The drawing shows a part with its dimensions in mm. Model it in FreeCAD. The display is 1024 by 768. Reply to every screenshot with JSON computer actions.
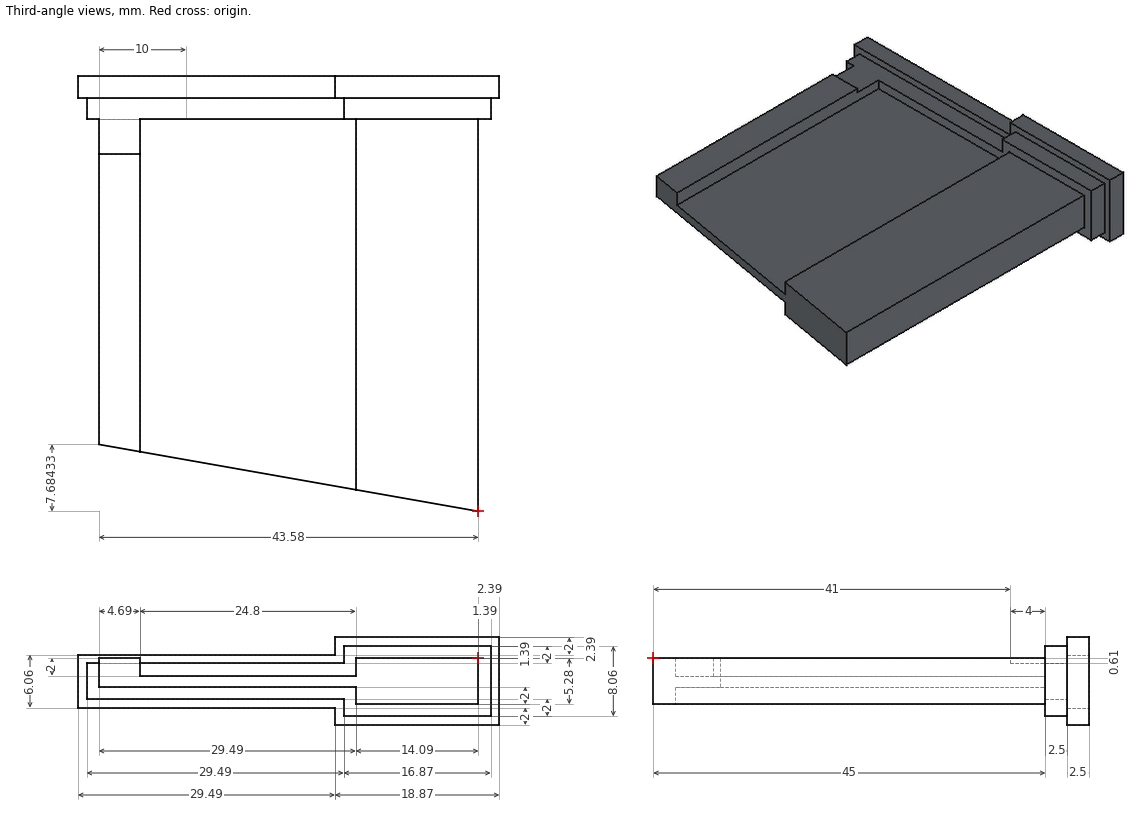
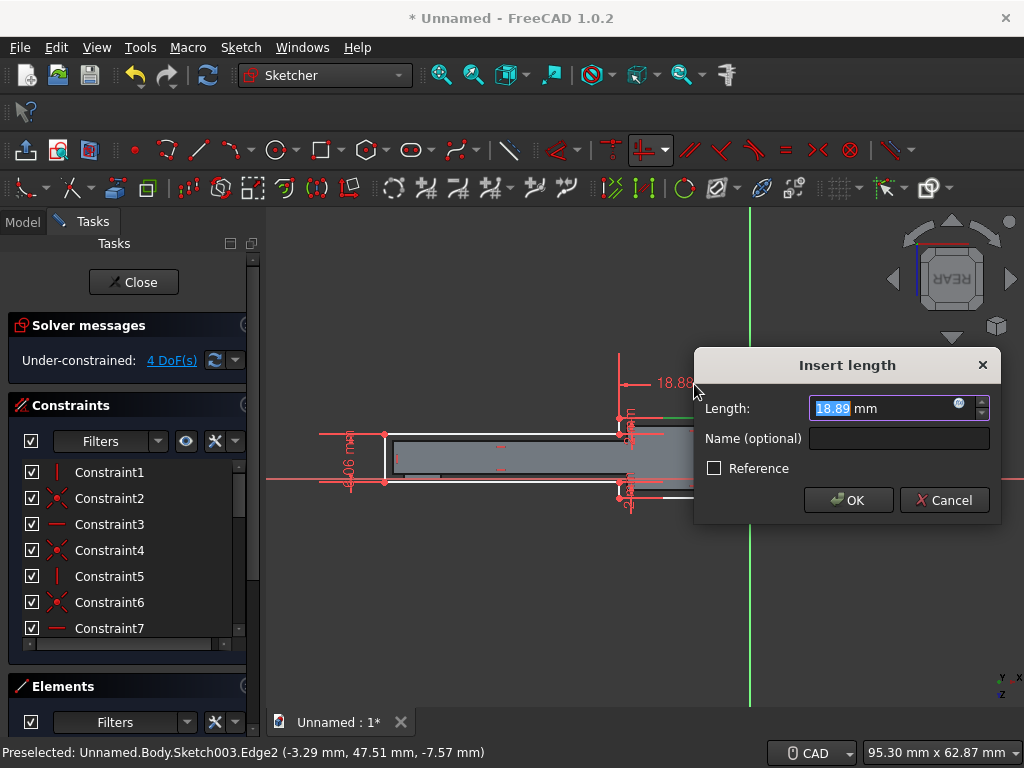
{"action": "type", "text": "18.87"}
{"action": "key", "text": "Return"}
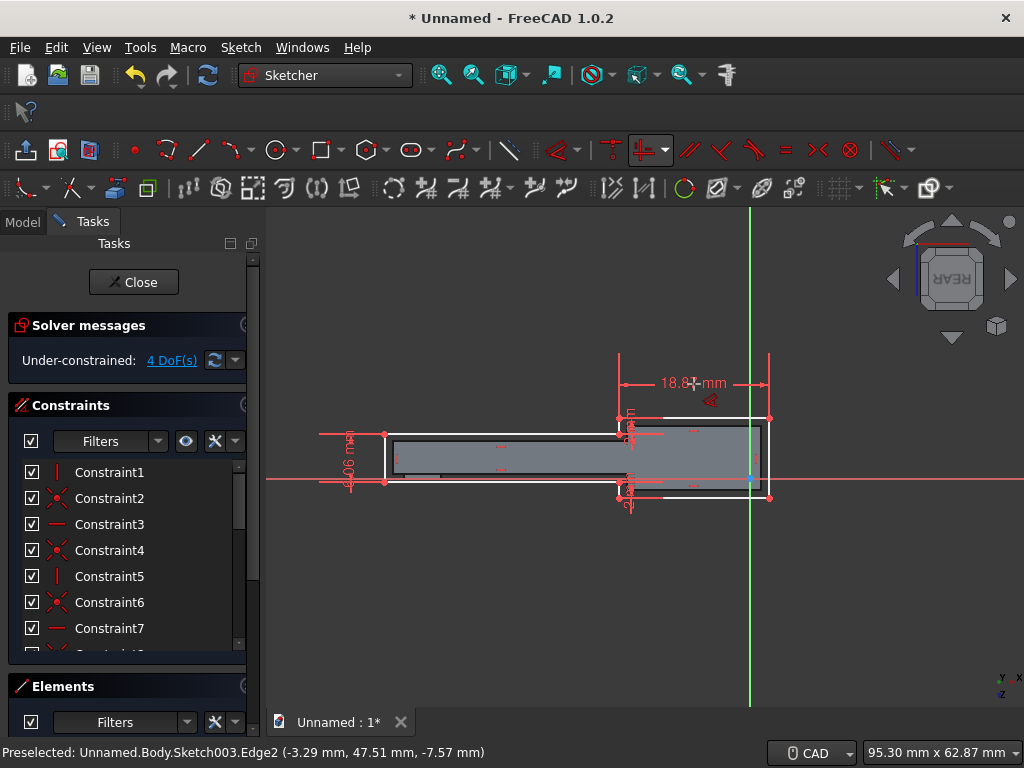
{"action": "left_click", "coordinate": [549, 434]}
{"action": "left_click", "coordinate": [502, 400]}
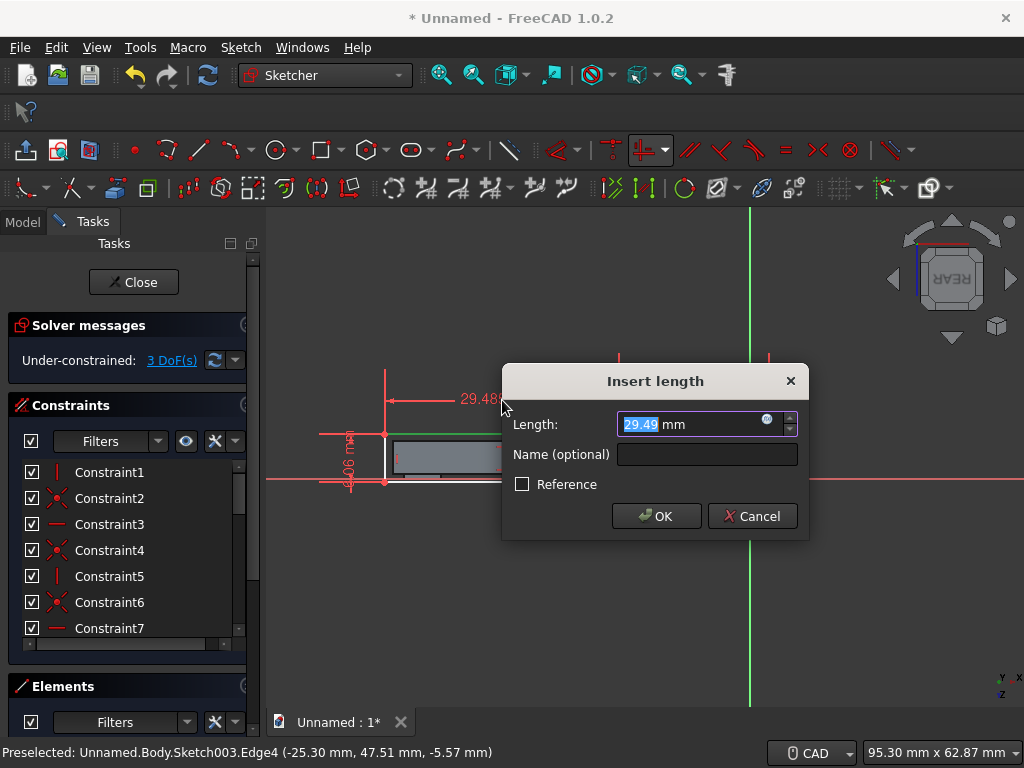
{"action": "type", "text": "29.49"}
{"action": "key", "text": "Return"}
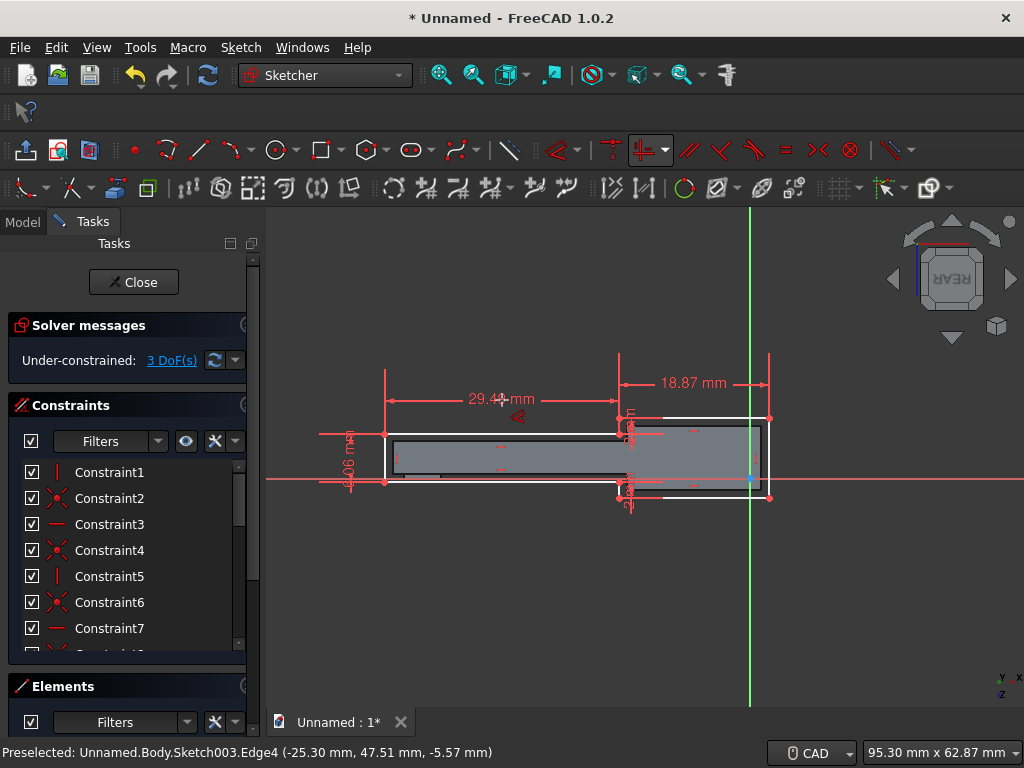
{"action": "left_click", "coordinate": [455, 482]}
{"action": "left_click", "coordinate": [502, 516]}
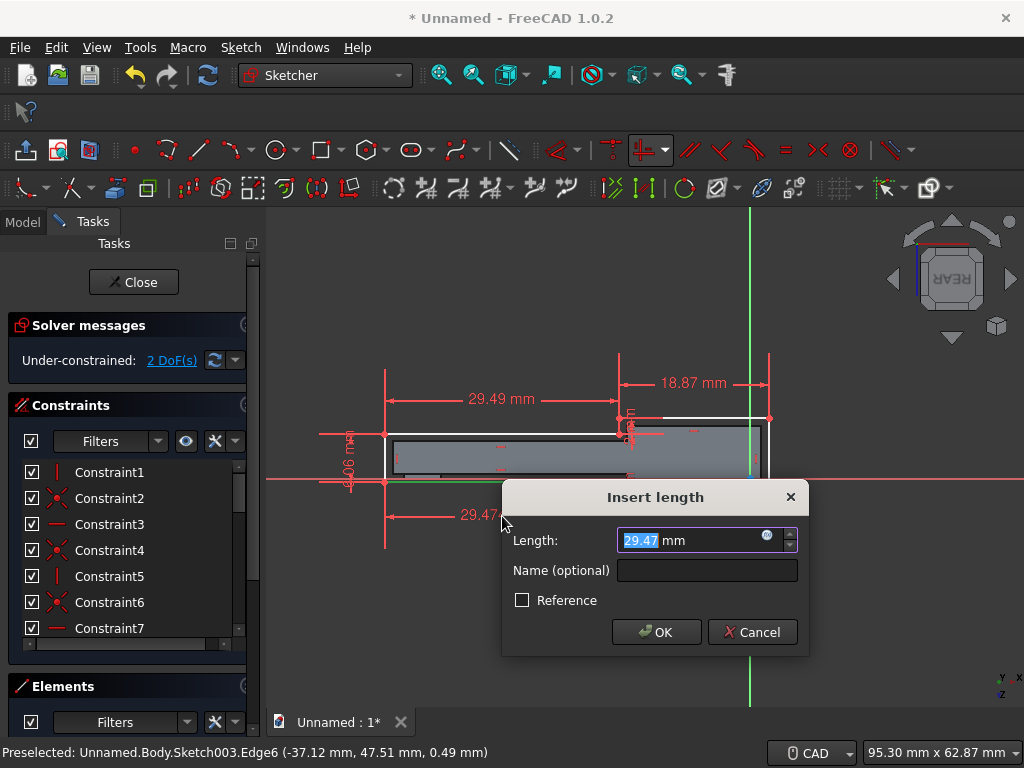
{"action": "type", "text": "29.49"}
{"action": "key", "text": "Return"}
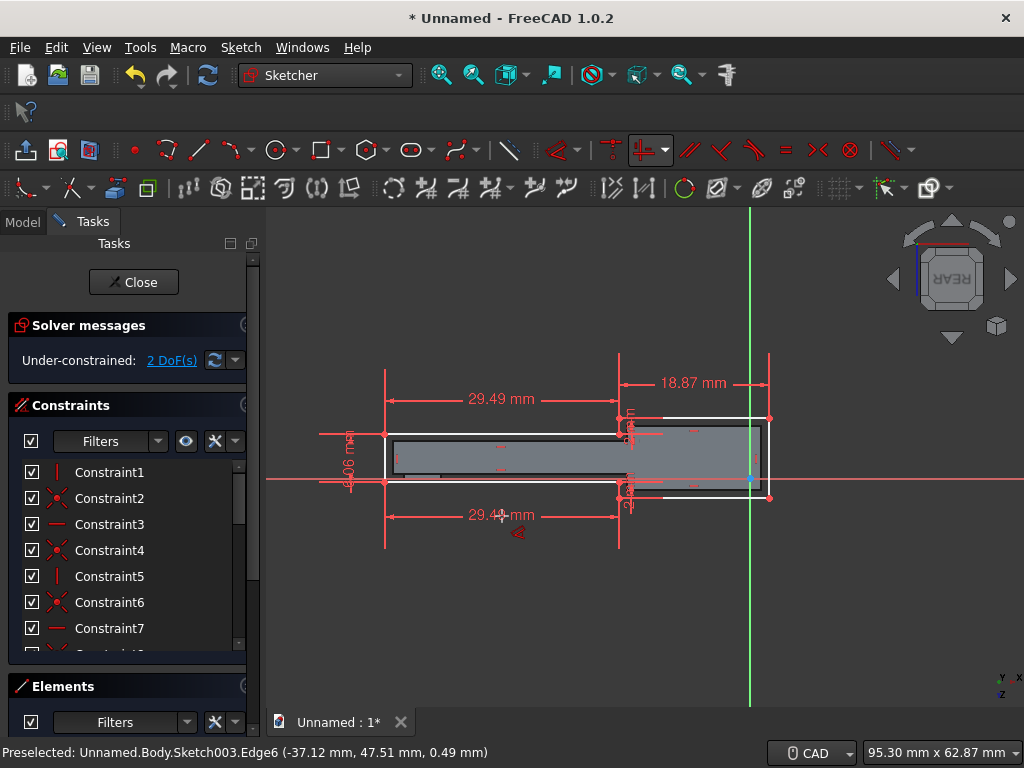
{"action": "scroll", "coordinate": [769, 498], "scroll_direction": "up", "scroll_amount": 4}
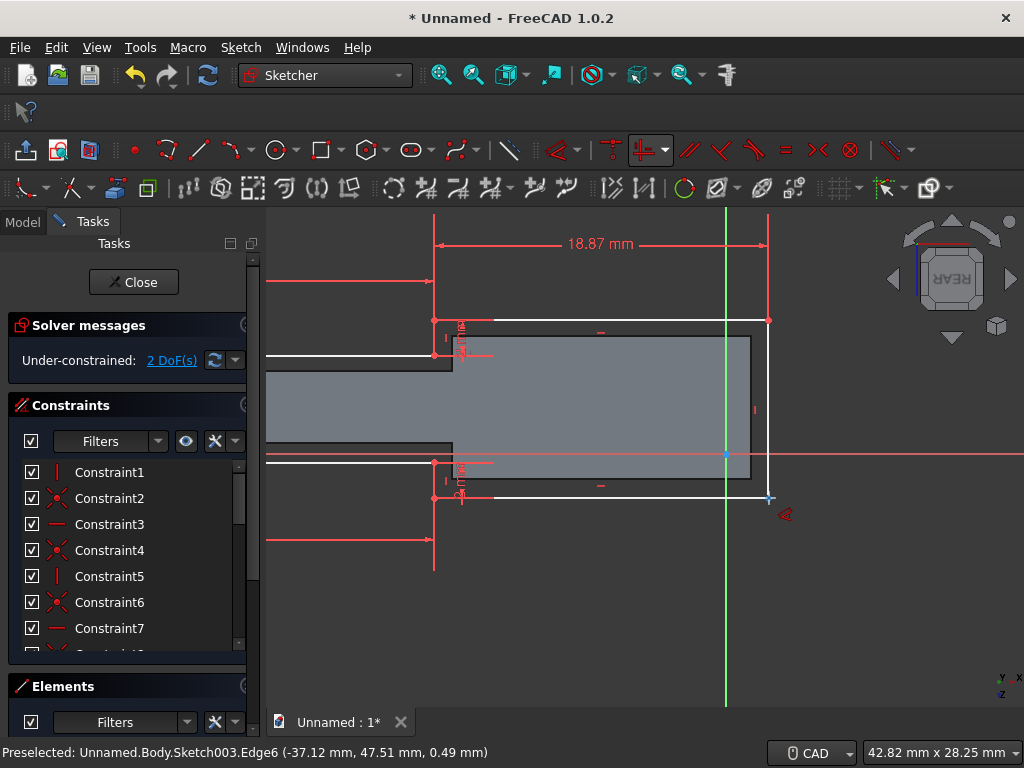
{"action": "left_click", "coordinate": [768, 498]}
{"action": "left_click", "coordinate": [747, 532]}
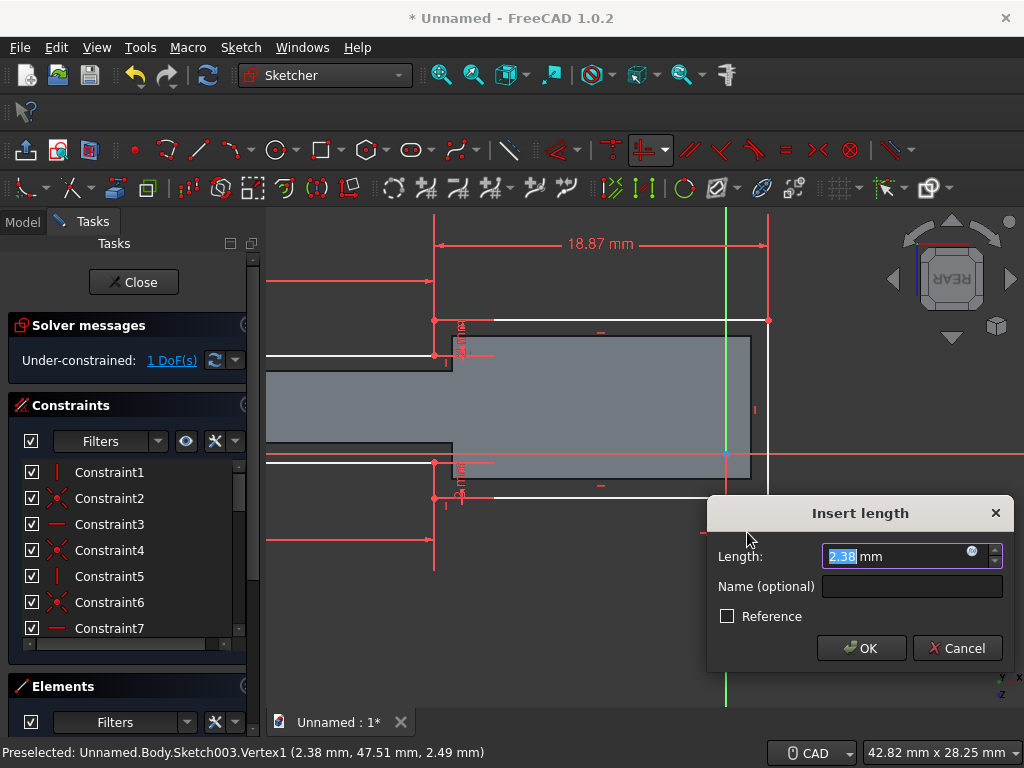
{"action": "type", "text": "2.39"}
{"action": "key", "text": "Return"}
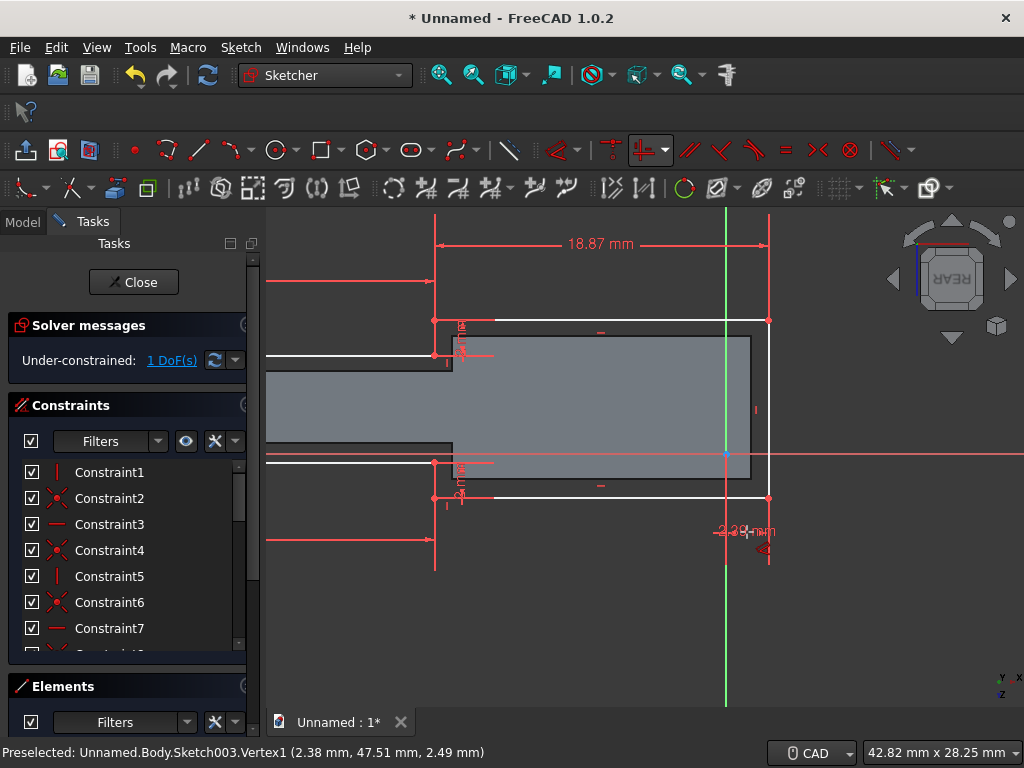
{"action": "left_click", "coordinate": [769, 498]}
{"action": "left_click", "coordinate": [803, 476]}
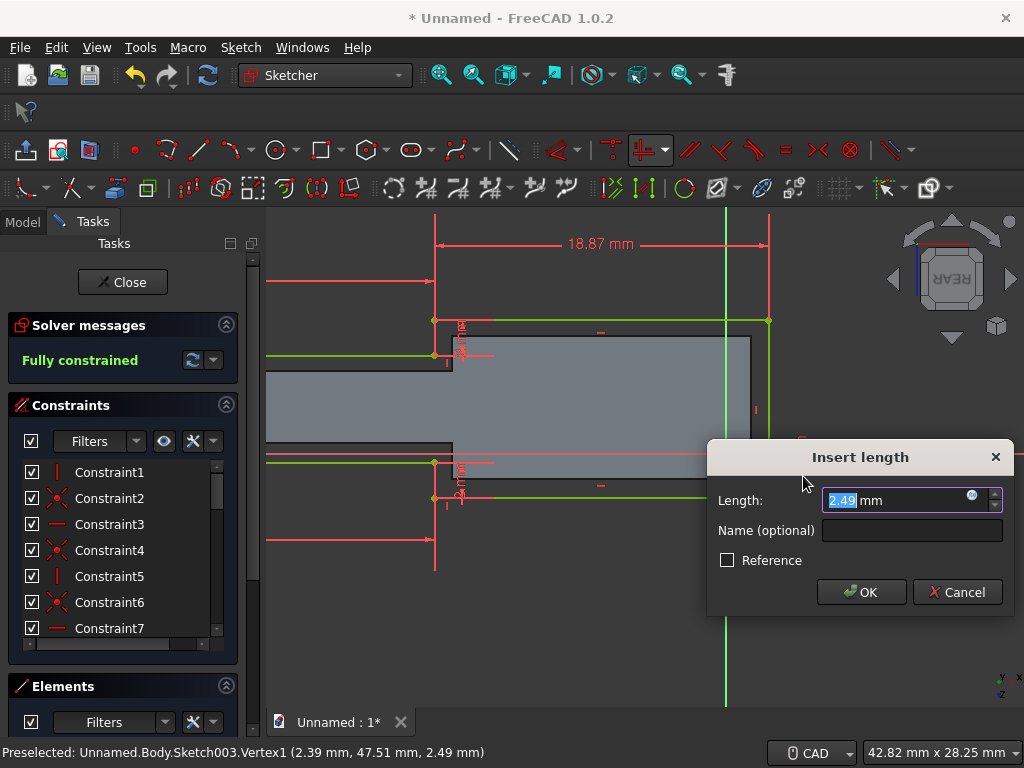
{"action": "type", "text": "2.39"}
{"action": "key", "text": "Return"}
{"action": "key", "text": "Escape"}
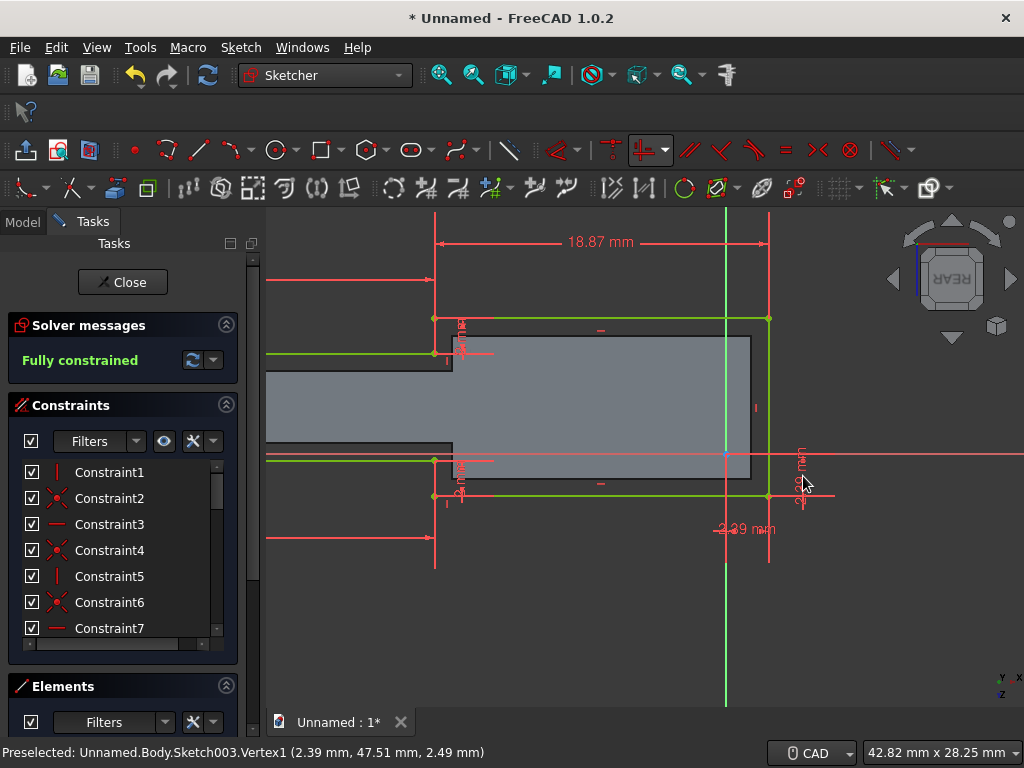
{"action": "left_click", "coordinate": [123, 282]}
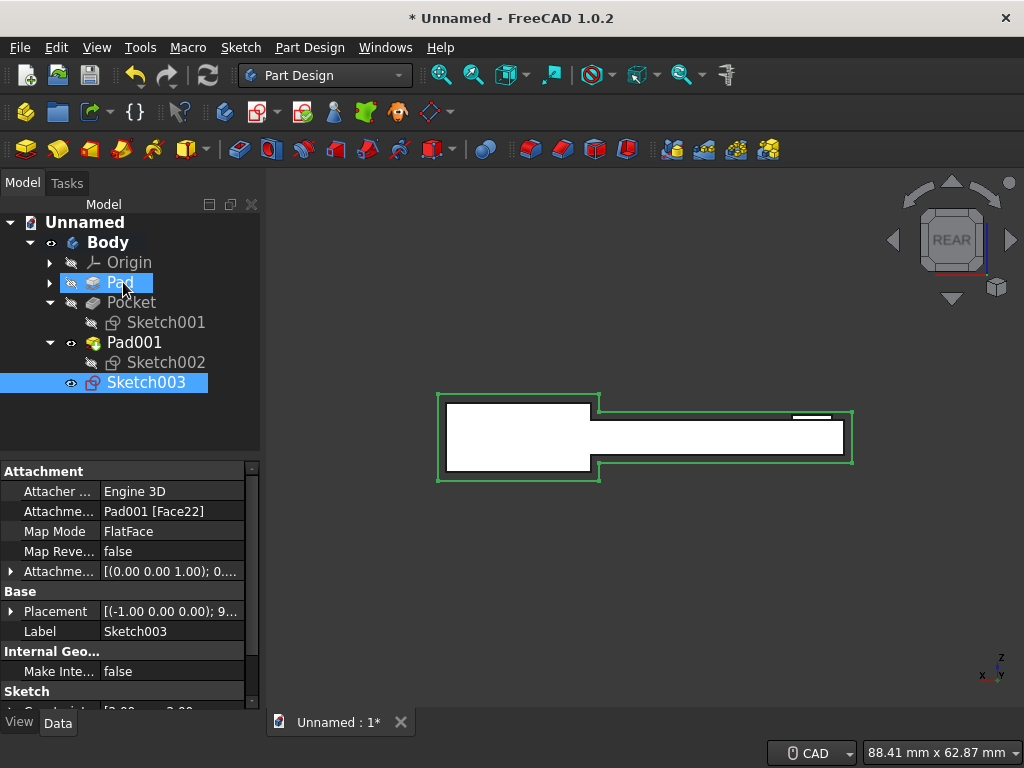
{"action": "left_click", "coordinate": [26, 150]}